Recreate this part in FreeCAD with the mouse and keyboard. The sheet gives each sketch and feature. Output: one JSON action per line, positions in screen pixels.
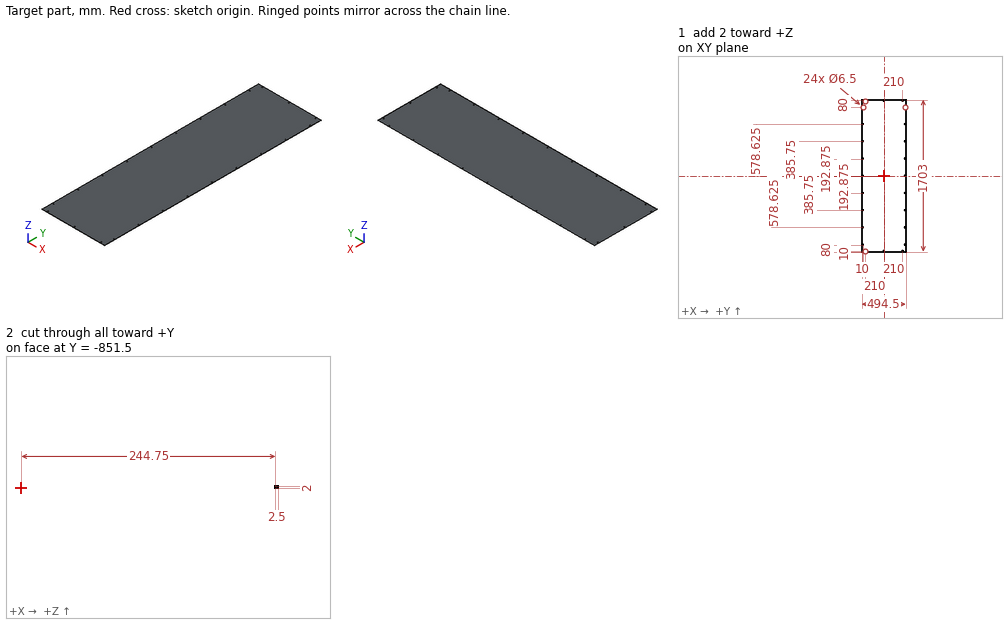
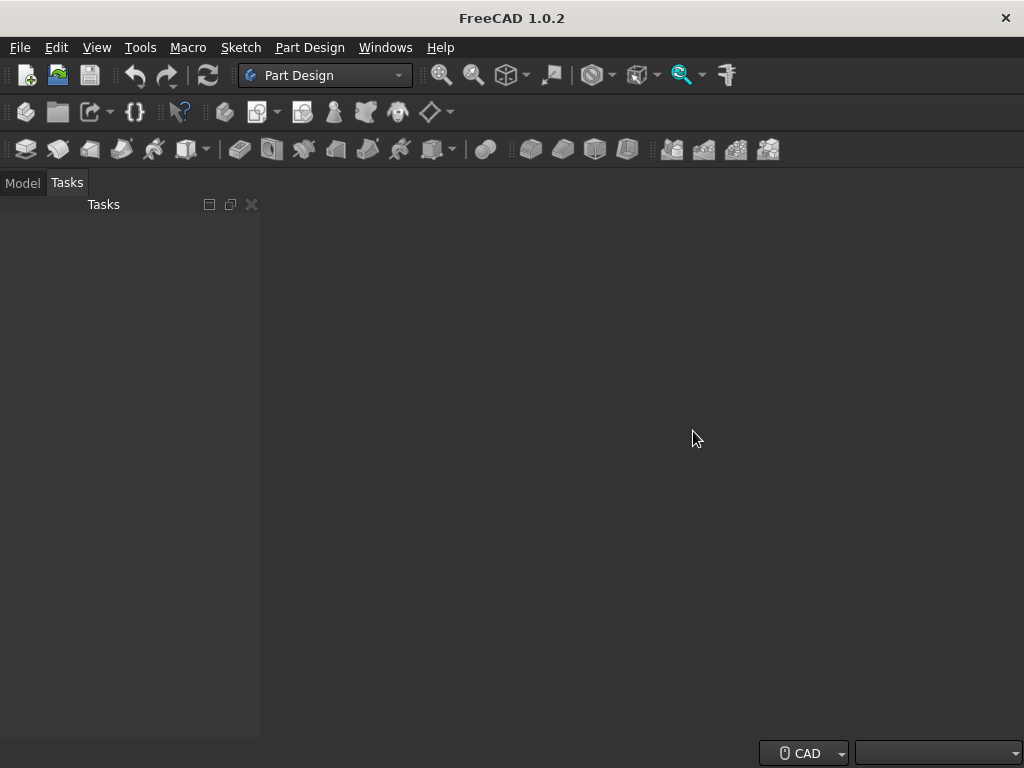
{"action": "left_click", "coordinate": [26, 76]}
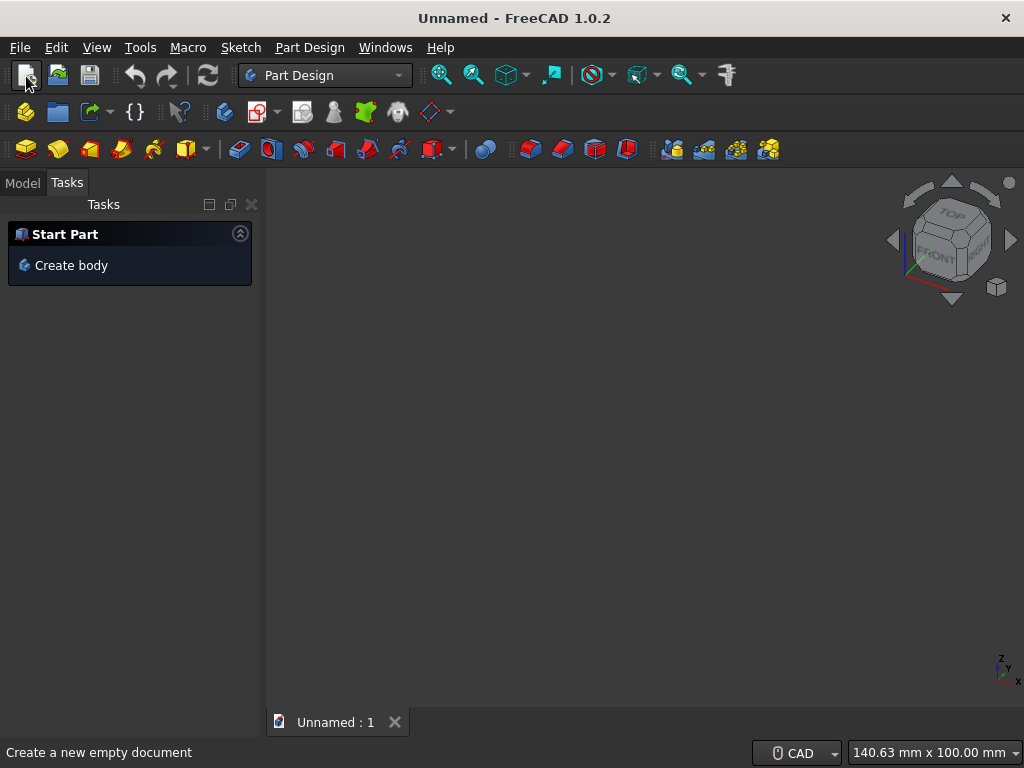
{"action": "left_click", "coordinate": [258, 112]}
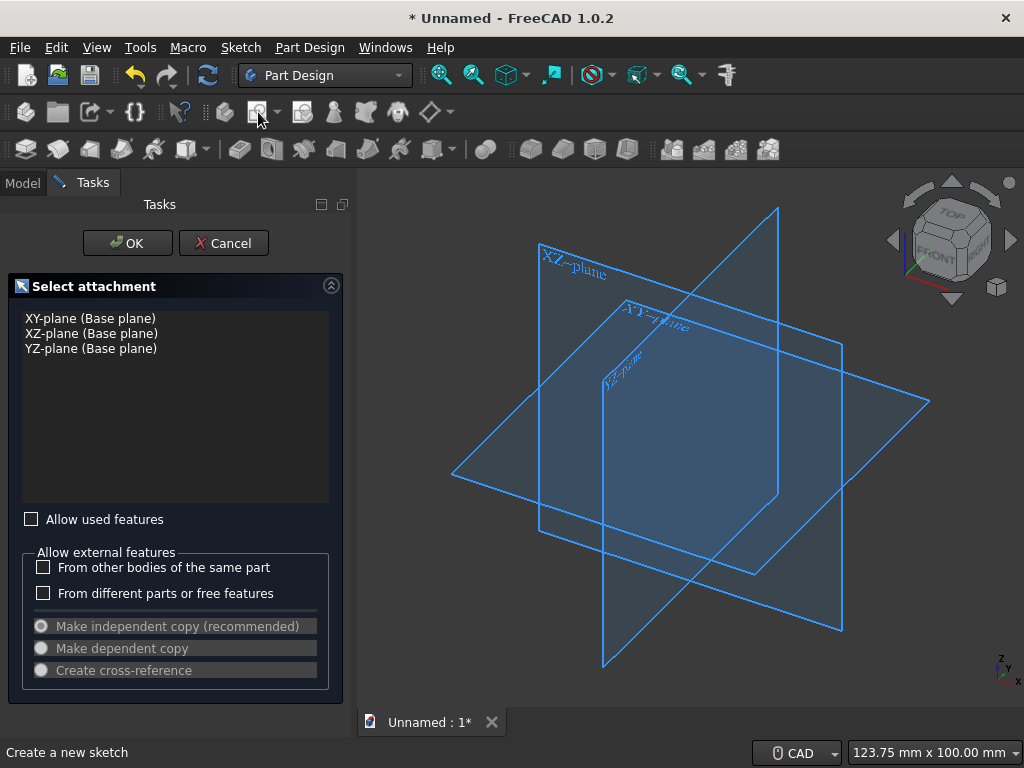
{"action": "left_click", "coordinate": [82, 318]}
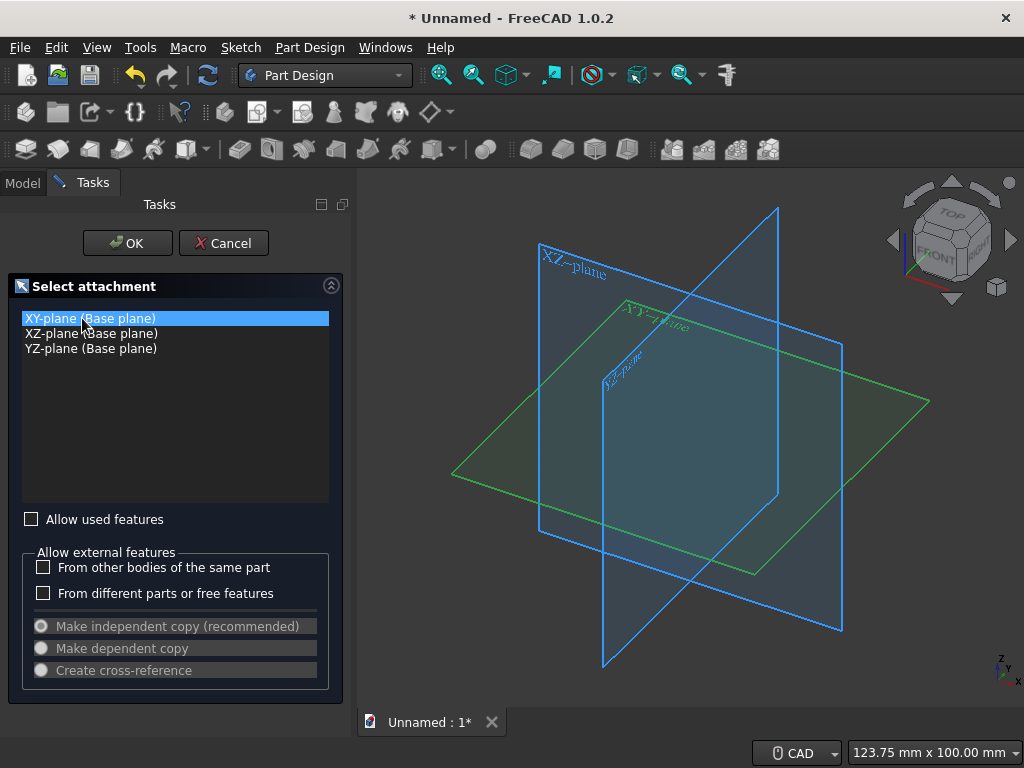
{"action": "left_click", "coordinate": [128, 243]}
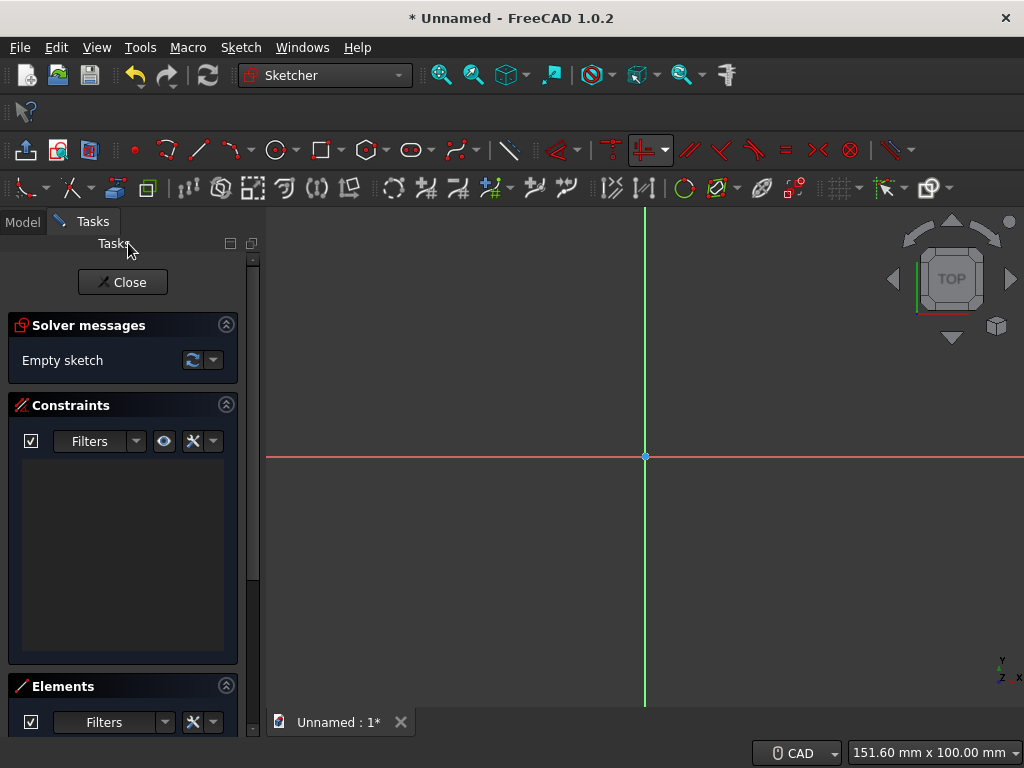
{"action": "scroll", "coordinate": [574, 457], "scroll_direction": "down", "scroll_amount": 16}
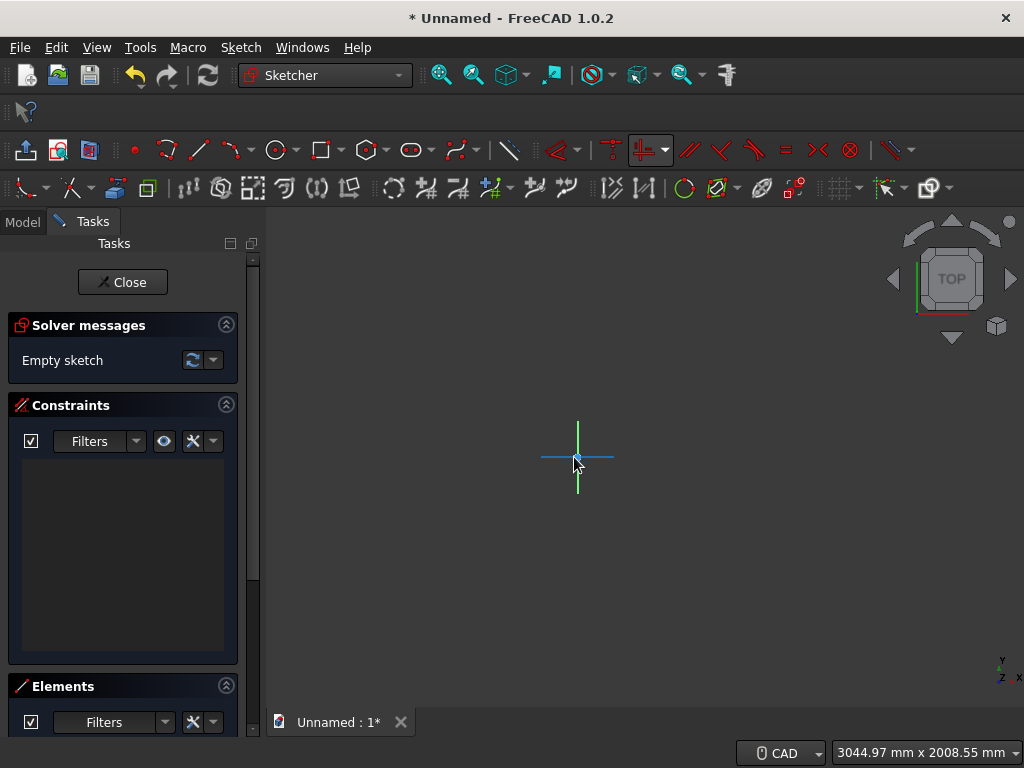
{"action": "left_click", "coordinate": [344, 150]}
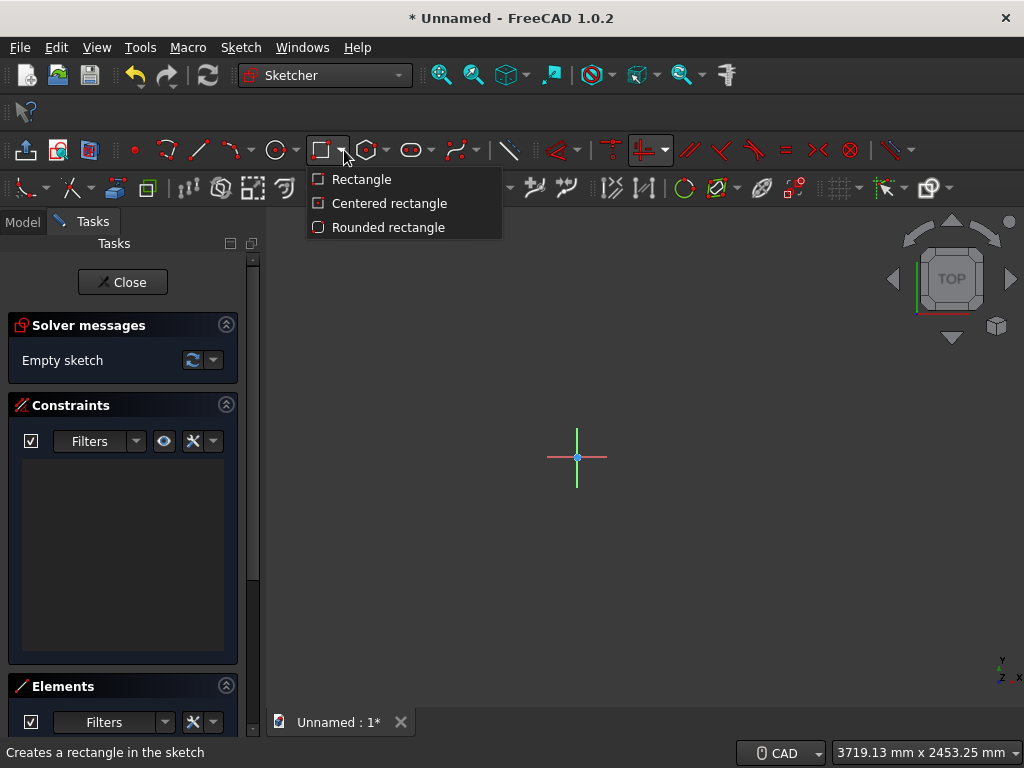
{"action": "left_click", "coordinate": [404, 203]}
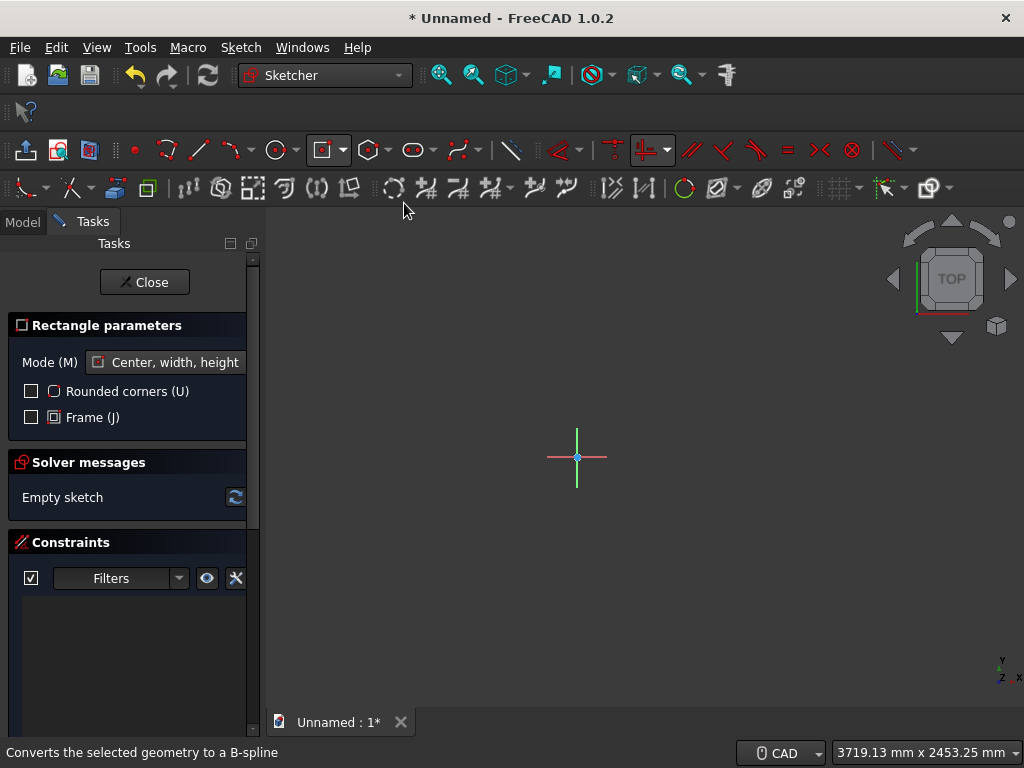
{"action": "left_click", "coordinate": [577, 457]}
{"action": "mouse_move", "coordinate": [628, 284]}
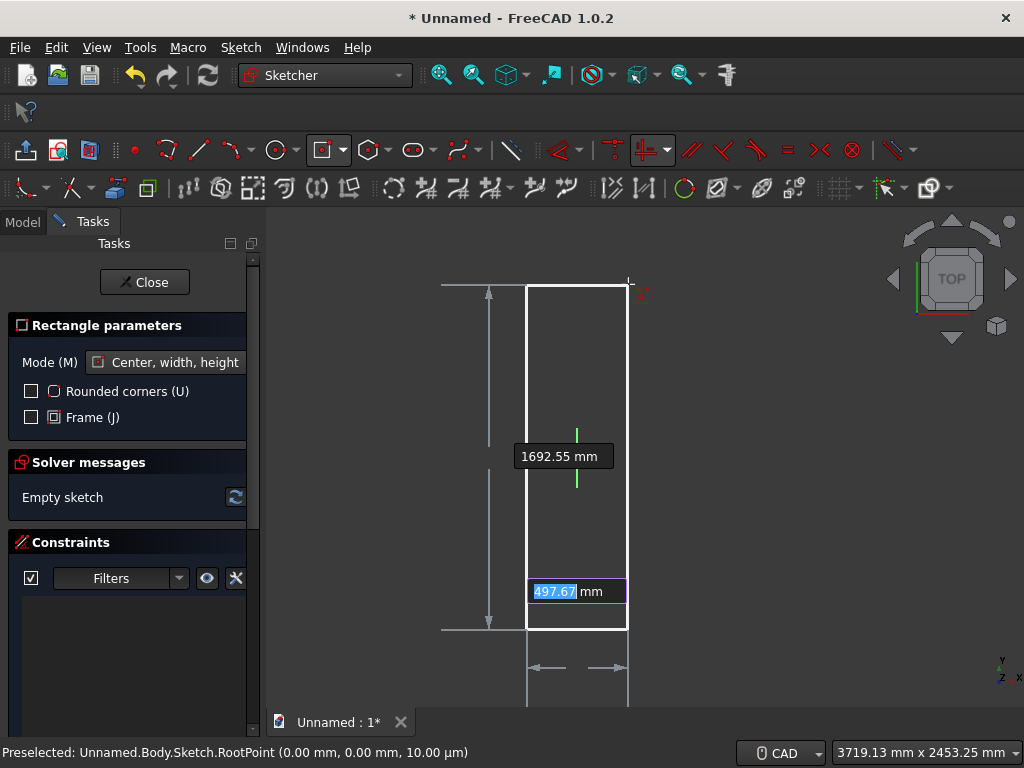
{"action": "type", "text": "494.5"}
{"action": "key", "text": "Tab"}
{"action": "type", "text": "1703"}
{"action": "key", "text": "Return"}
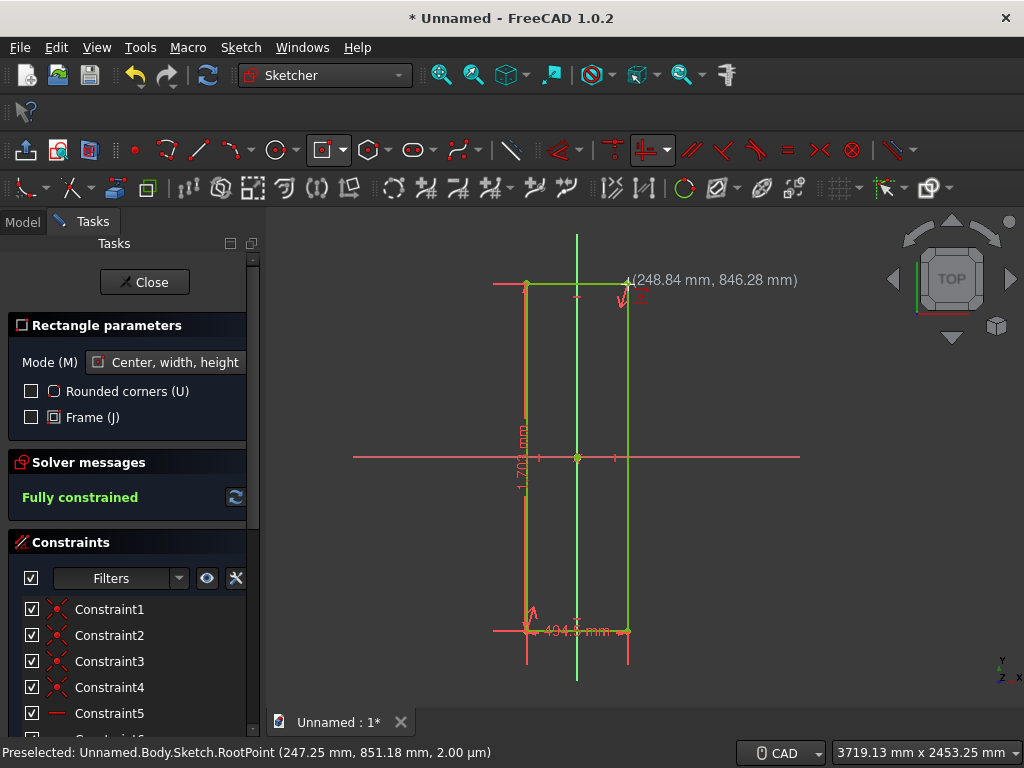
{"action": "left_click", "coordinate": [276, 150]}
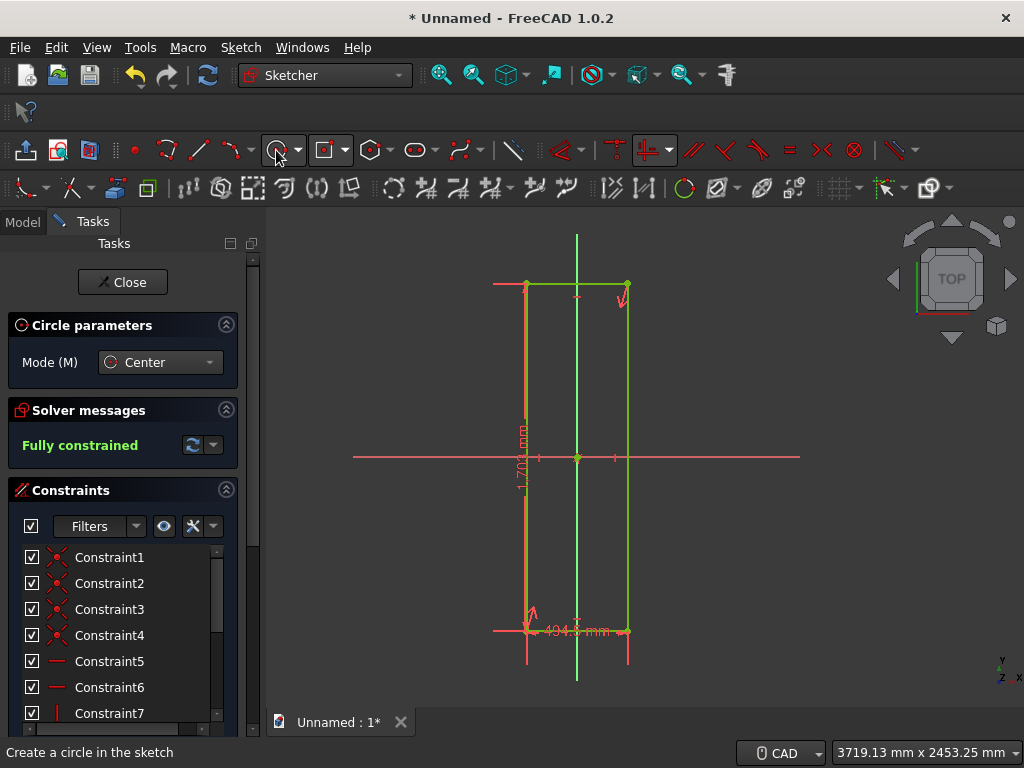
{"action": "scroll", "coordinate": [529, 615], "scroll_direction": "up", "scroll_amount": 18}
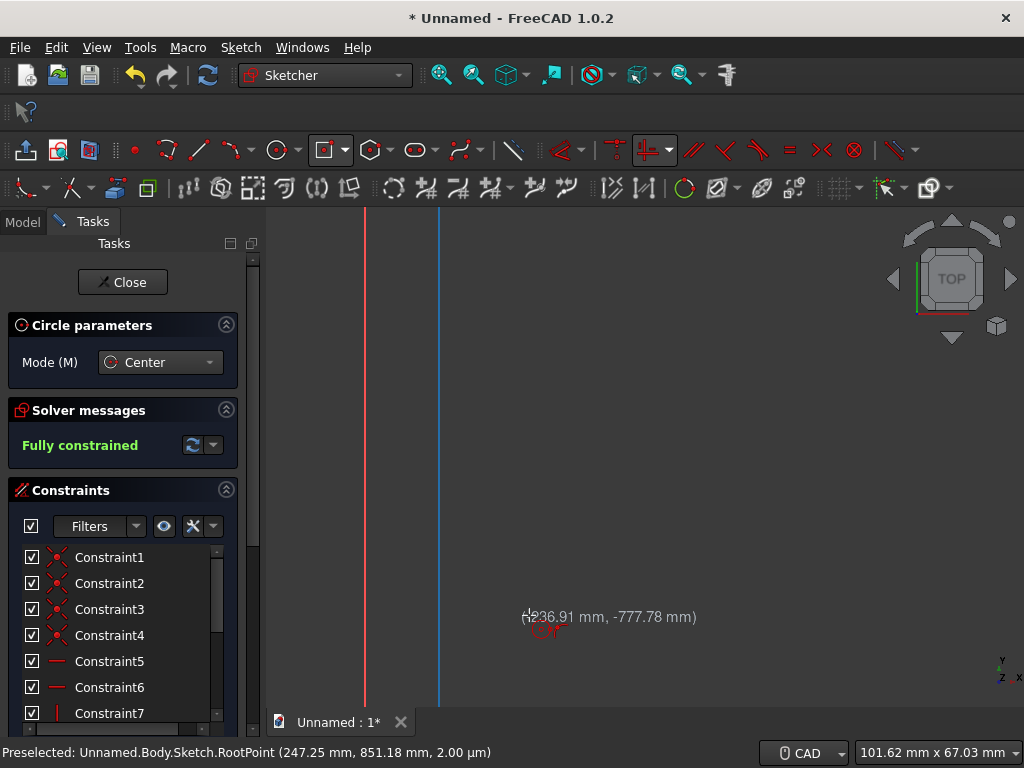
{"action": "scroll", "coordinate": [529, 615], "scroll_direction": "down", "scroll_amount": 18}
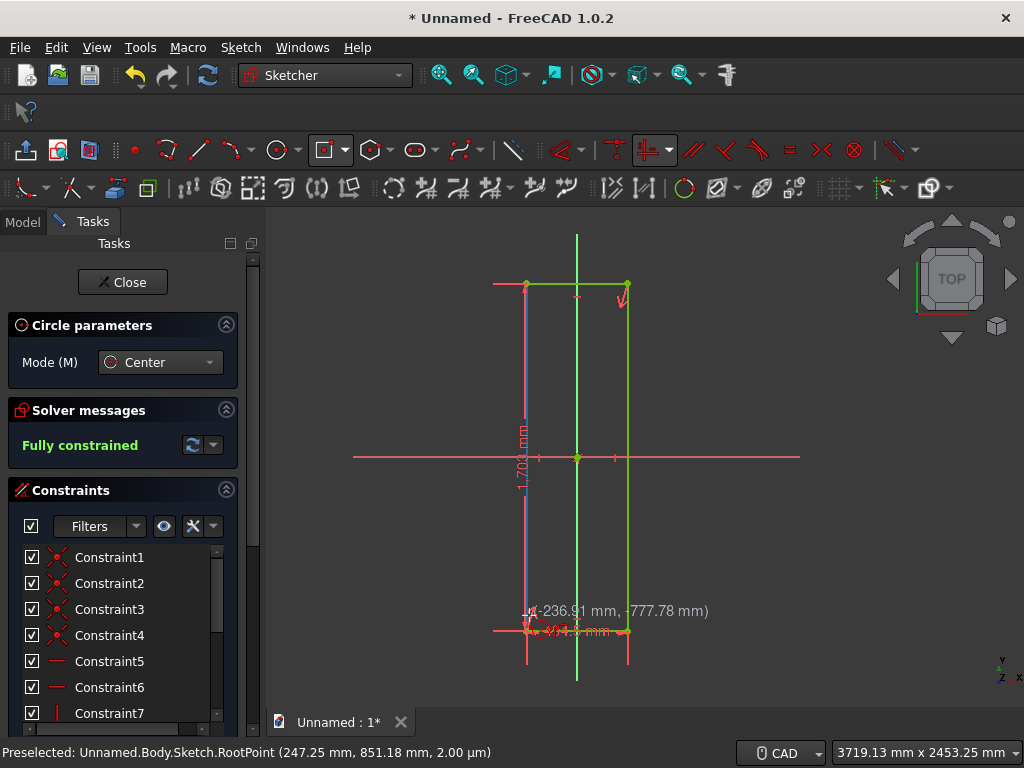
{"action": "scroll", "coordinate": [529, 615], "scroll_direction": "up", "scroll_amount": 11}